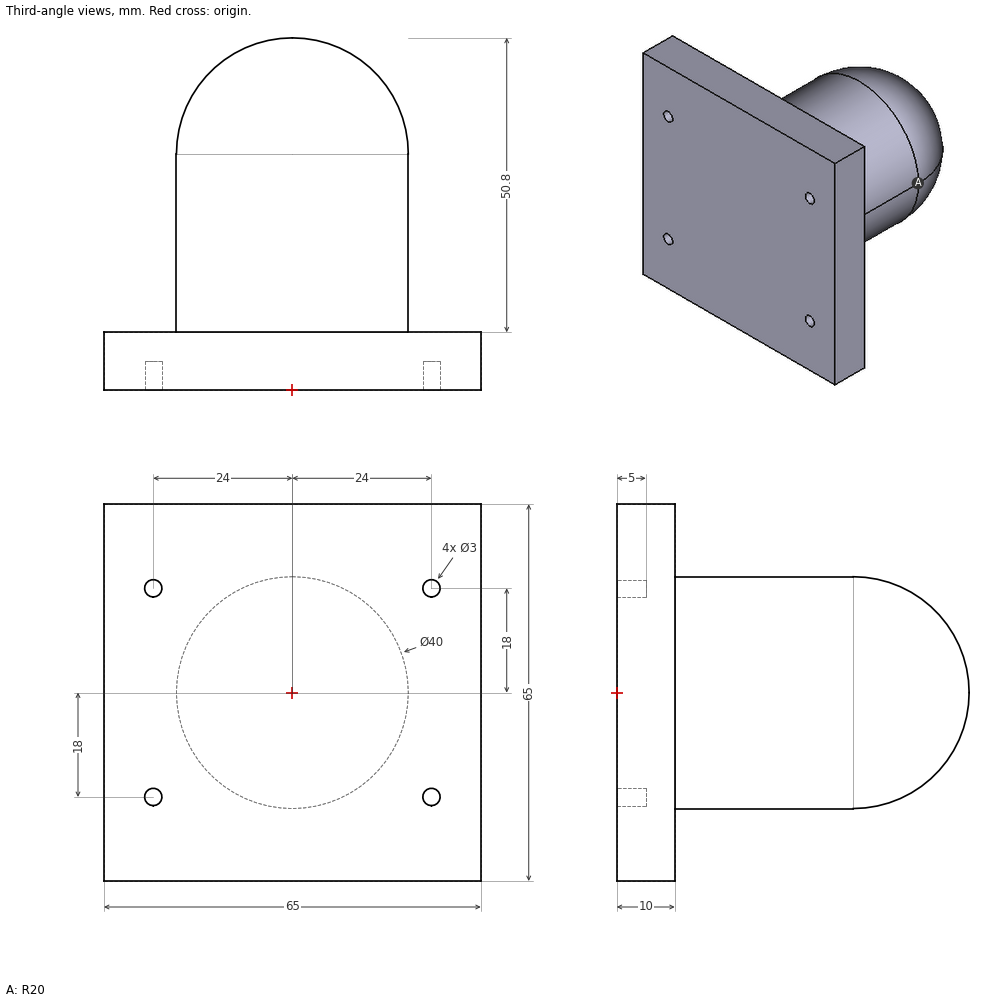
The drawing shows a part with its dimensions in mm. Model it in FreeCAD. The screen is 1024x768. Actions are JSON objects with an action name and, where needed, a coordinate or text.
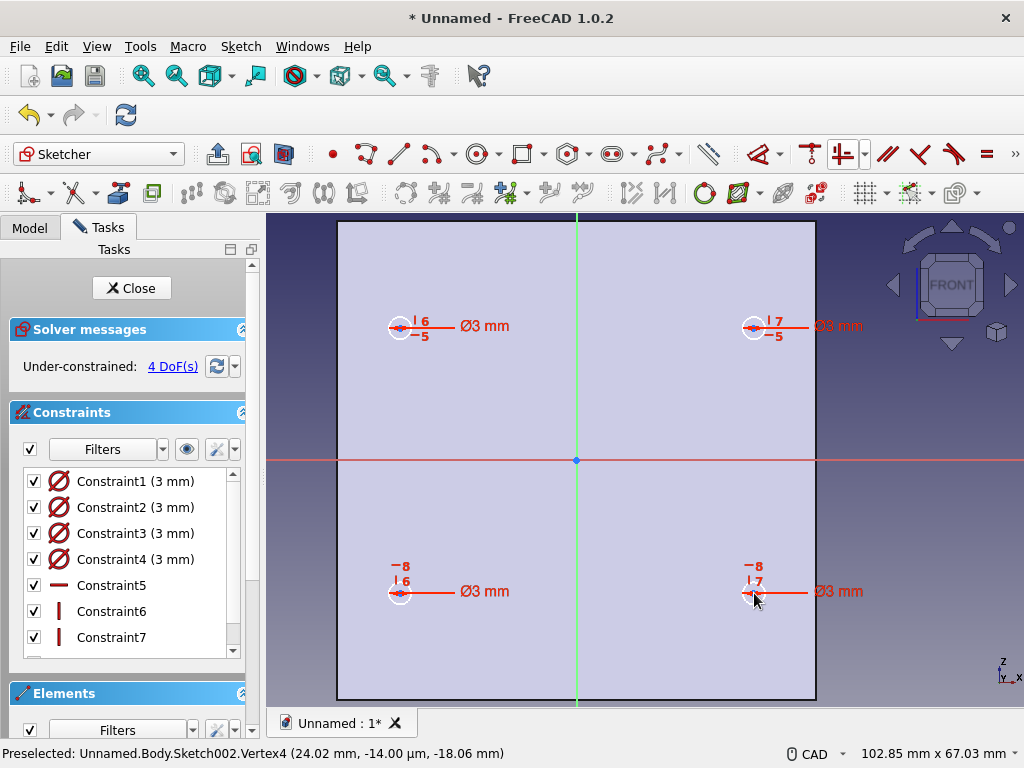
{"action": "left_click", "coordinate": [754, 328]}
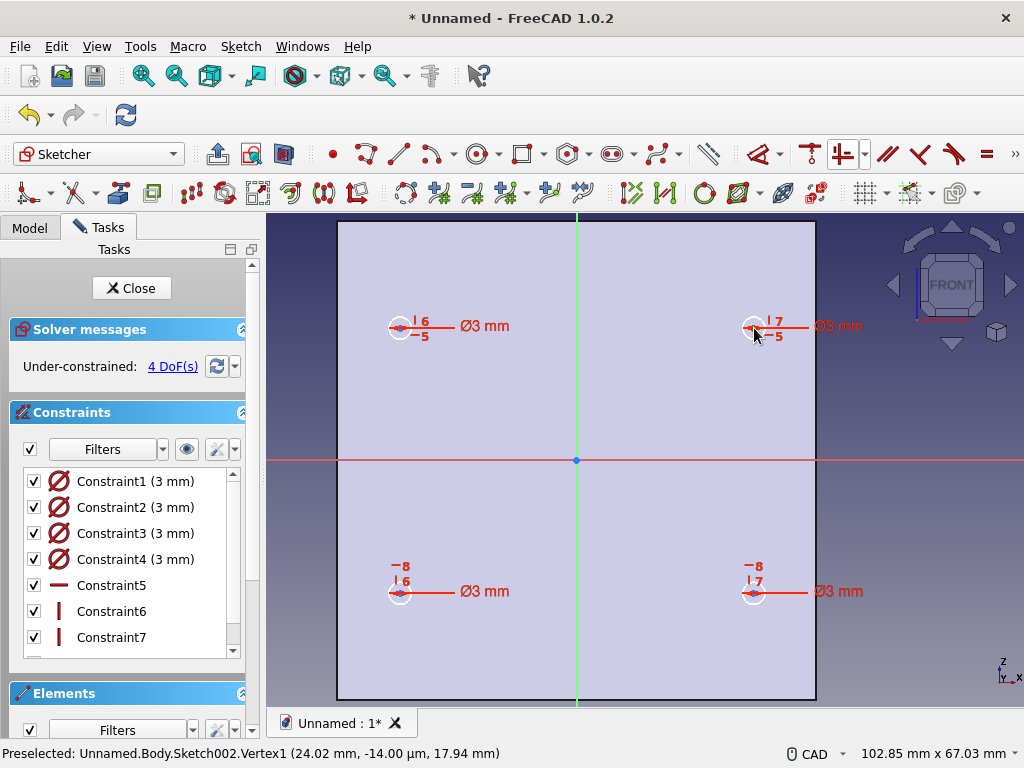
{"action": "left_click", "coordinate": [780, 154]}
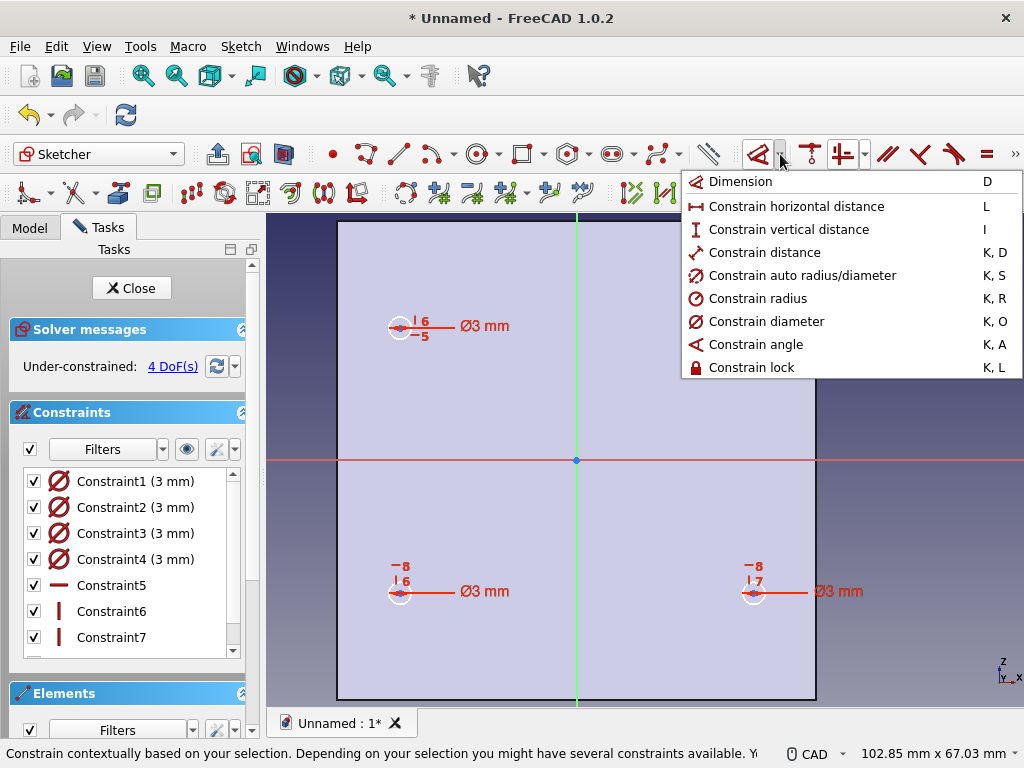
{"action": "left_click", "coordinate": [852, 206]}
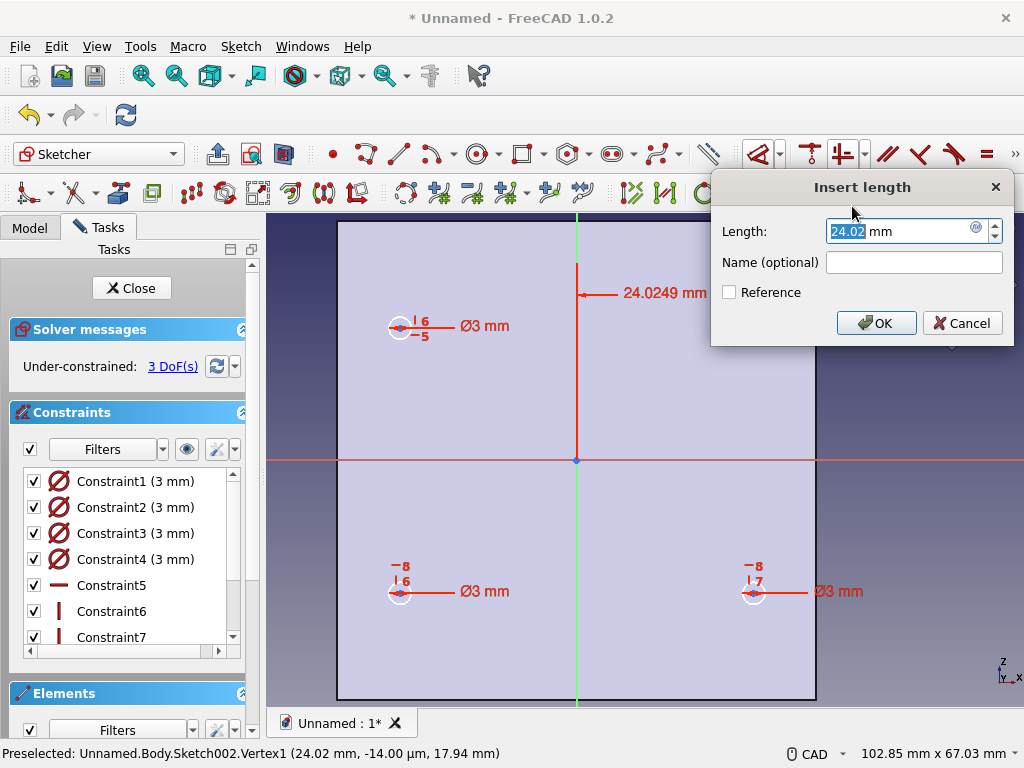
{"action": "type", "text": "24"}
{"action": "key", "text": "Return"}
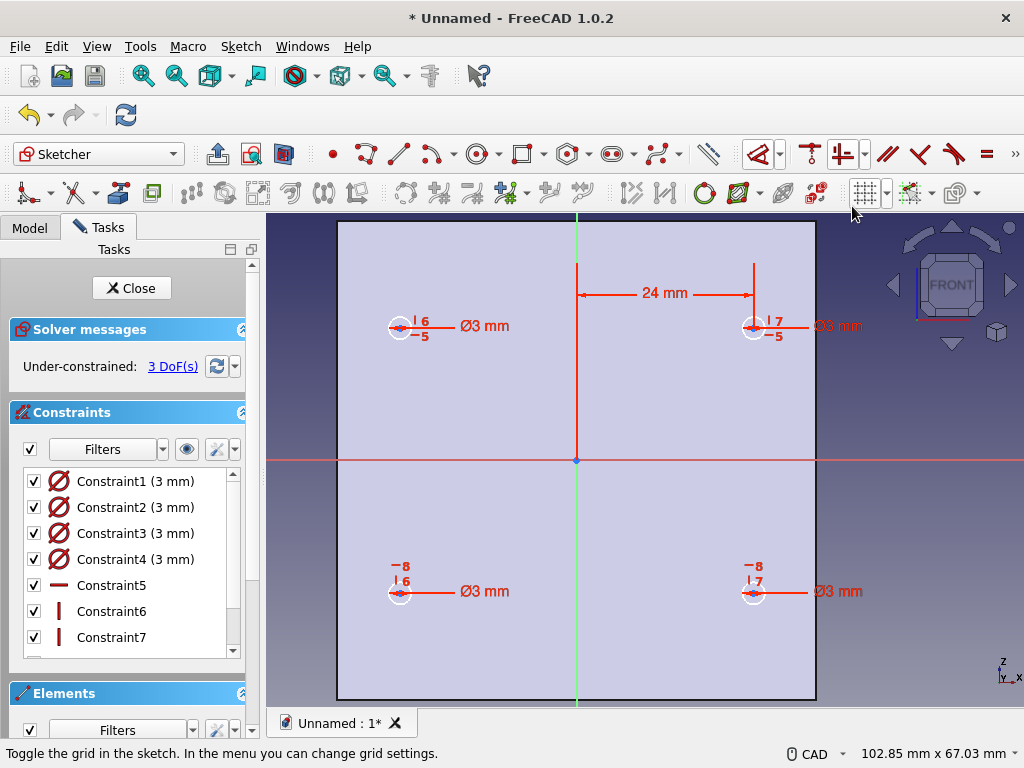
{"action": "left_click", "coordinate": [754, 328]}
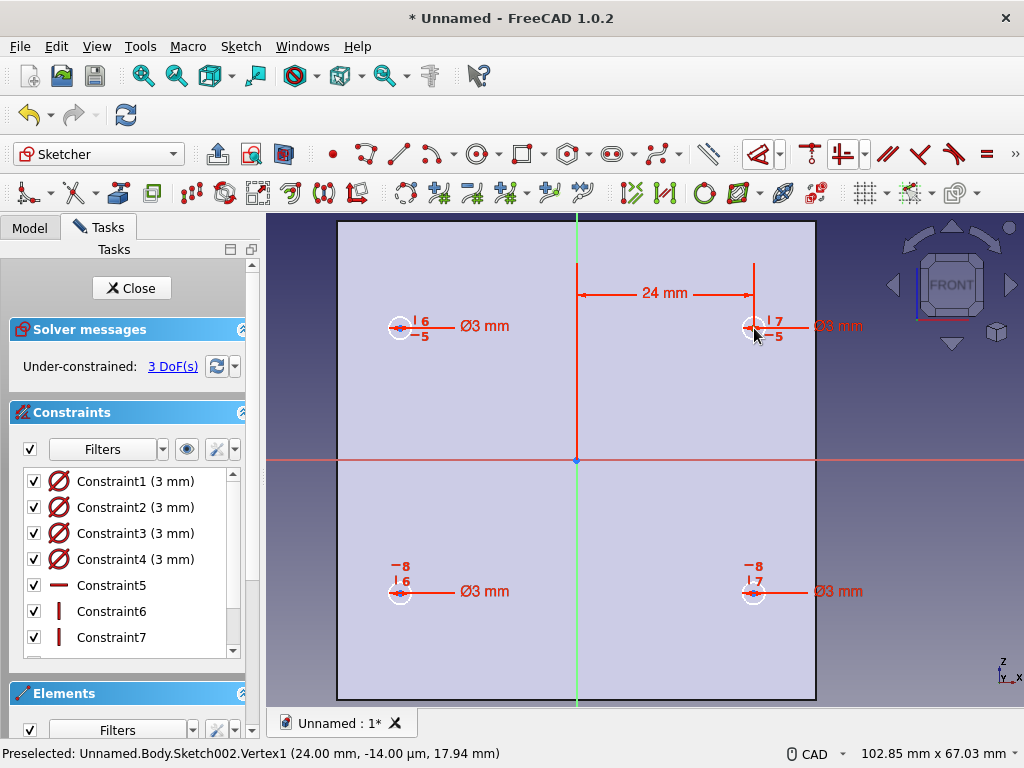
{"action": "left_click", "coordinate": [780, 154]}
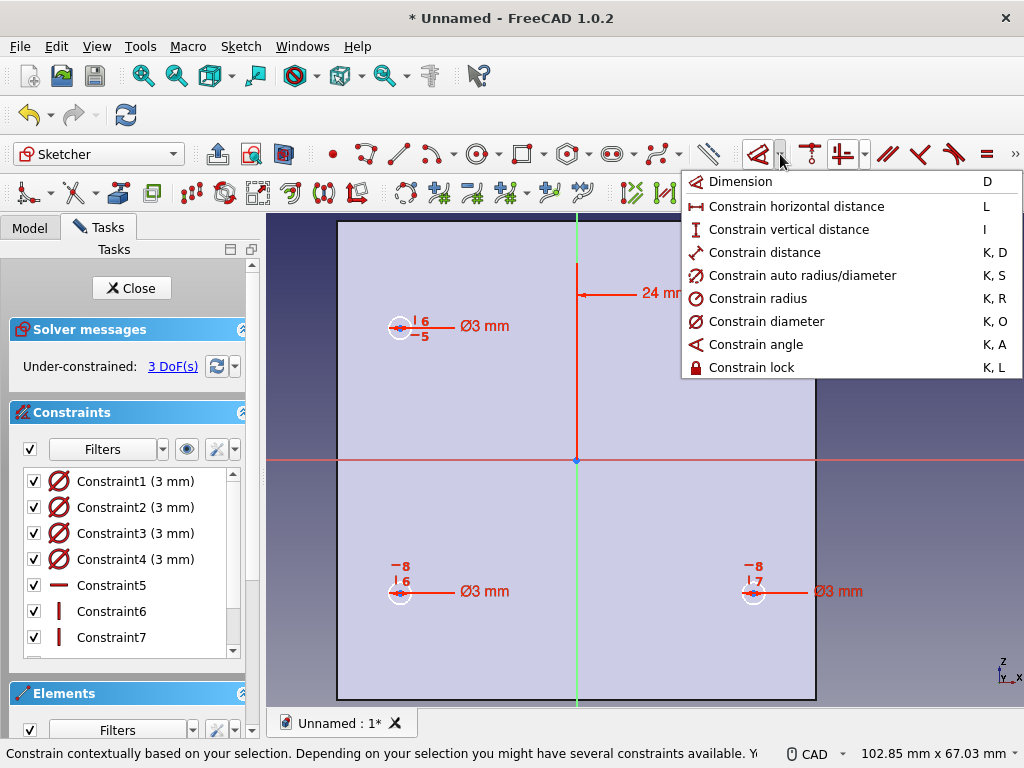
{"action": "left_click", "coordinate": [852, 230]}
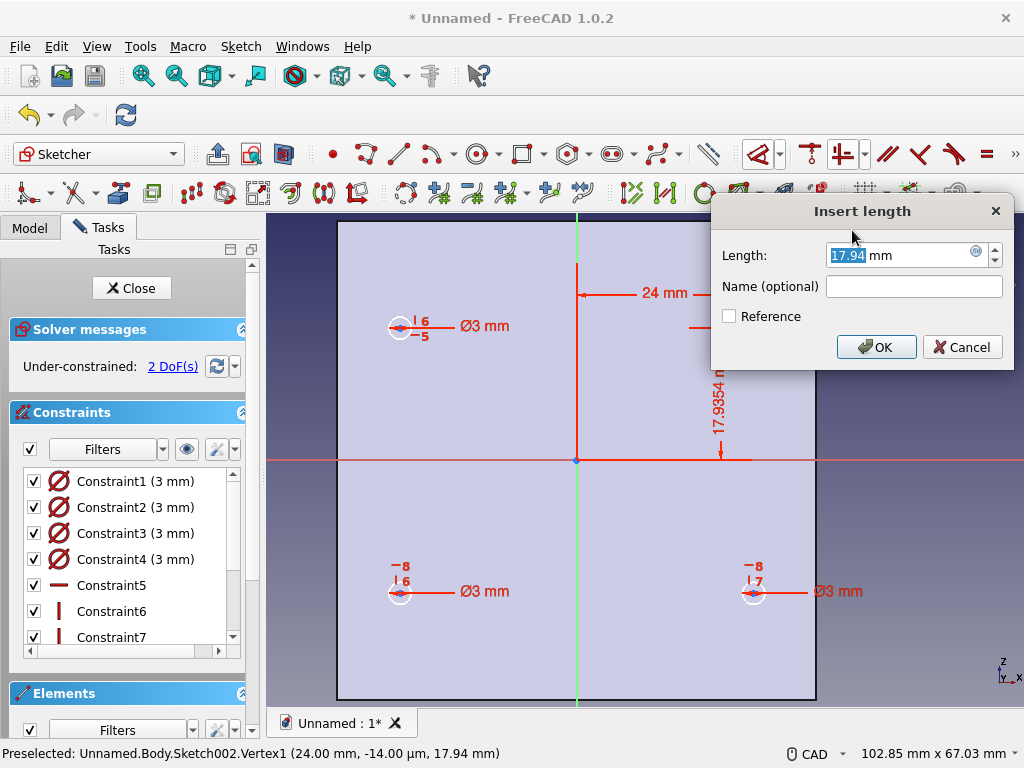
{"action": "type", "text": "18"}
{"action": "key", "text": "Return"}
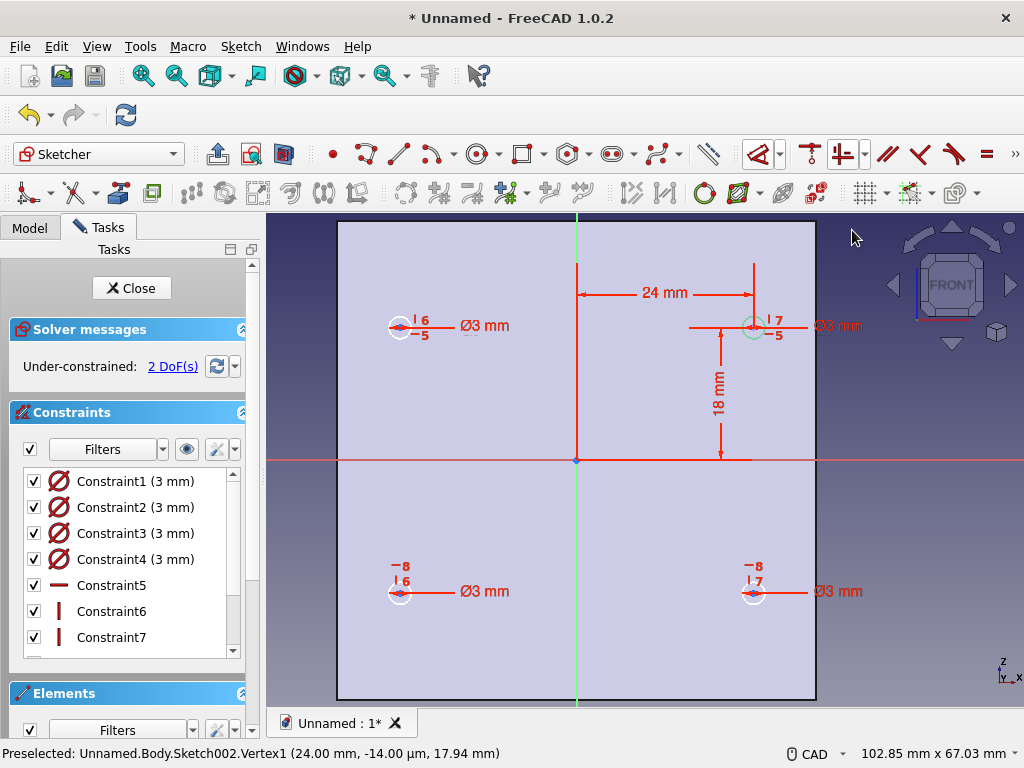
{"action": "left_click", "coordinate": [400, 328]}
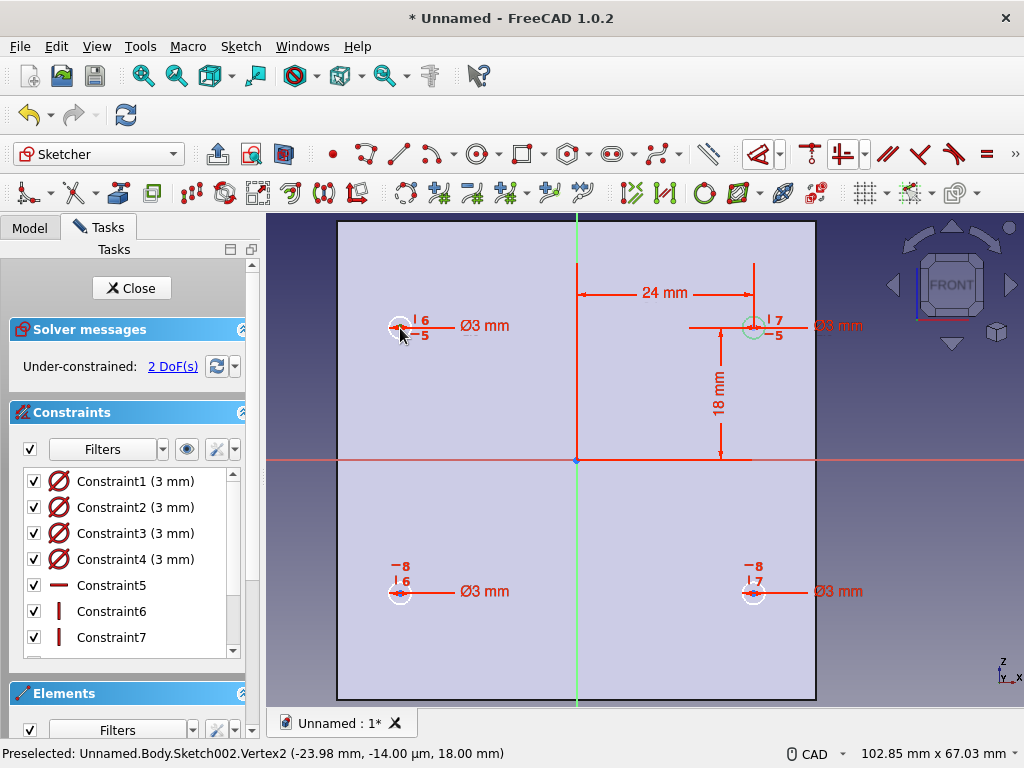
{"action": "key", "text": "l"}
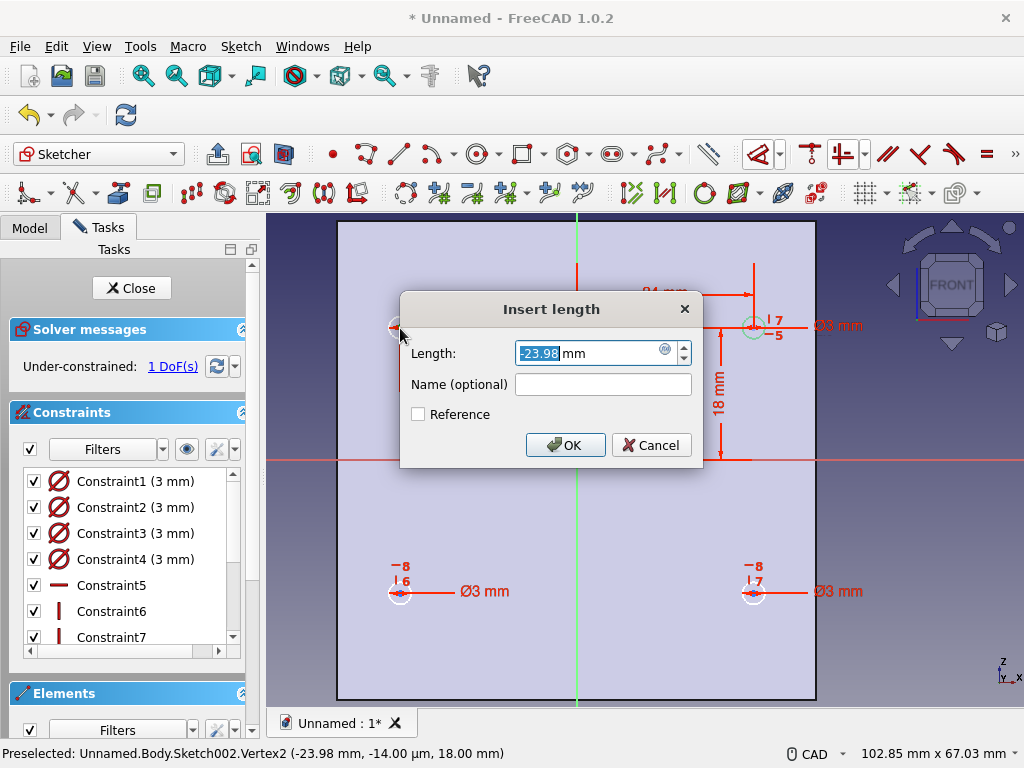
{"action": "type", "text": "-24"}
{"action": "key", "text": "Return"}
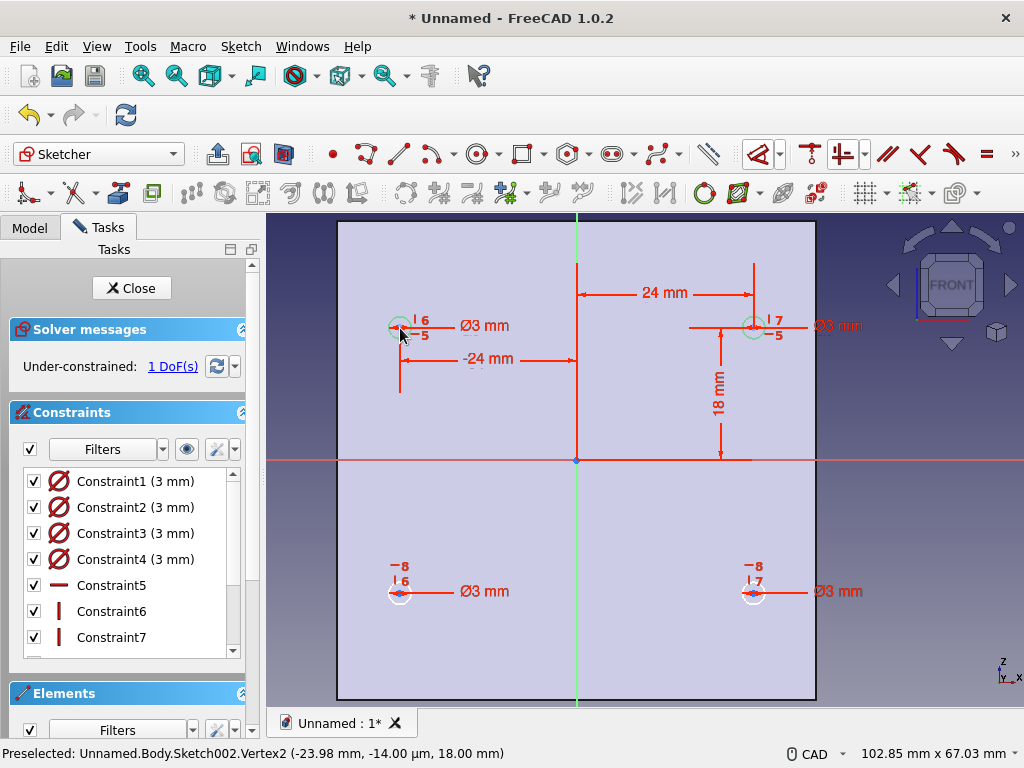
{"action": "left_click", "coordinate": [400, 593]}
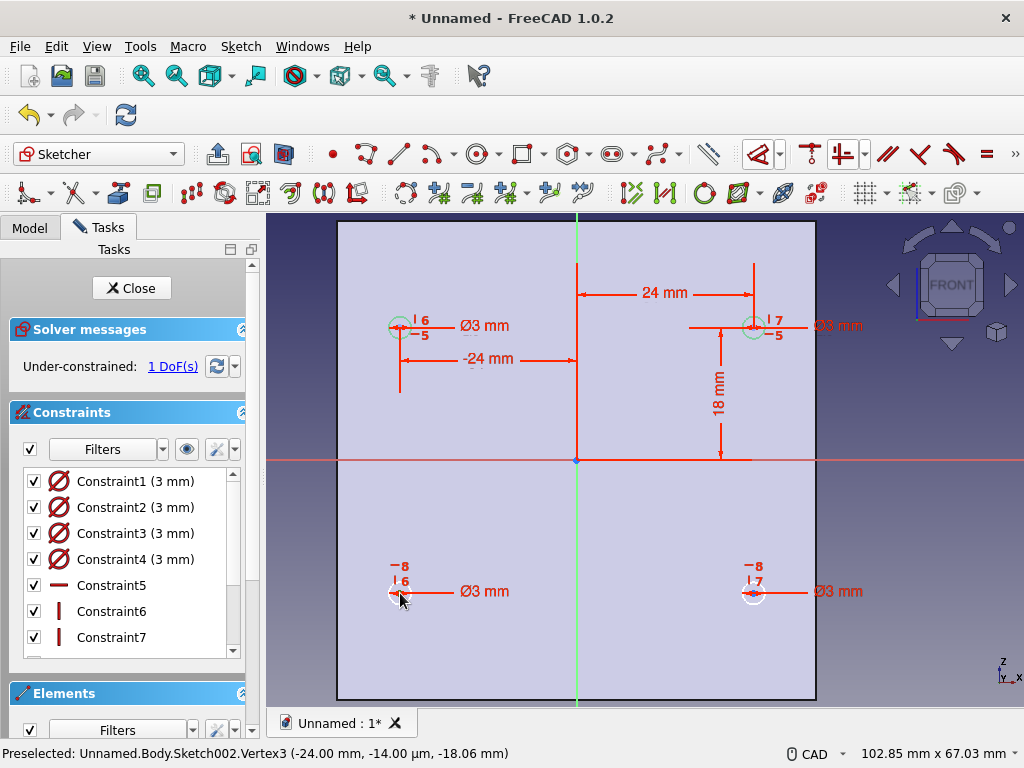
{"action": "left_click", "coordinate": [780, 154]}